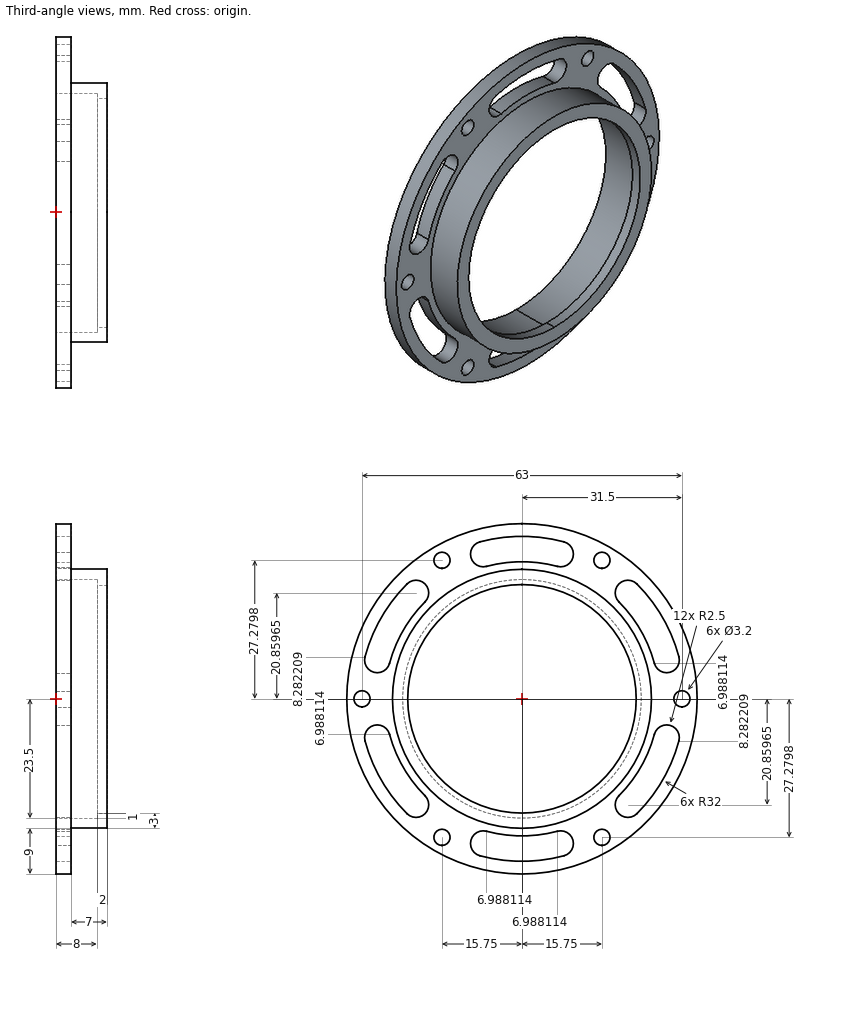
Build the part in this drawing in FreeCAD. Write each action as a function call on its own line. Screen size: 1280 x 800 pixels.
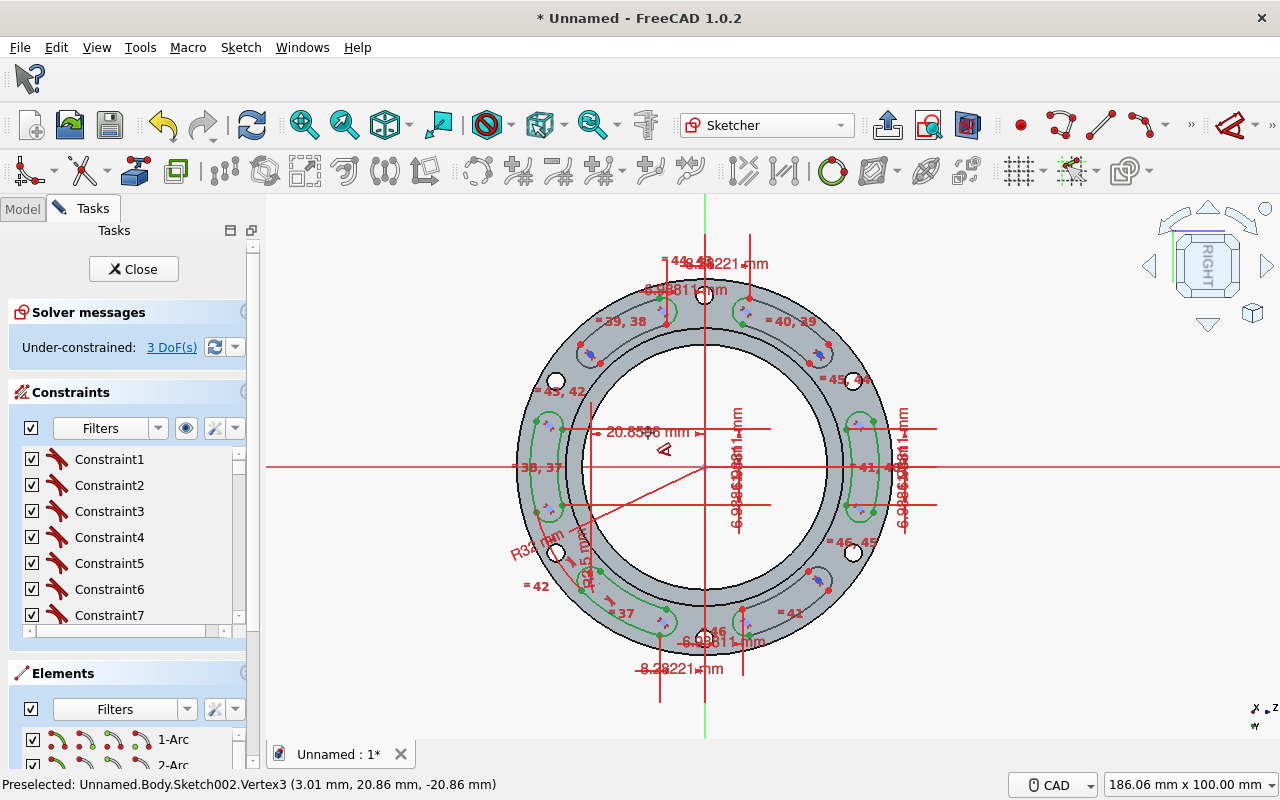
click(590, 354)
click(648, 501)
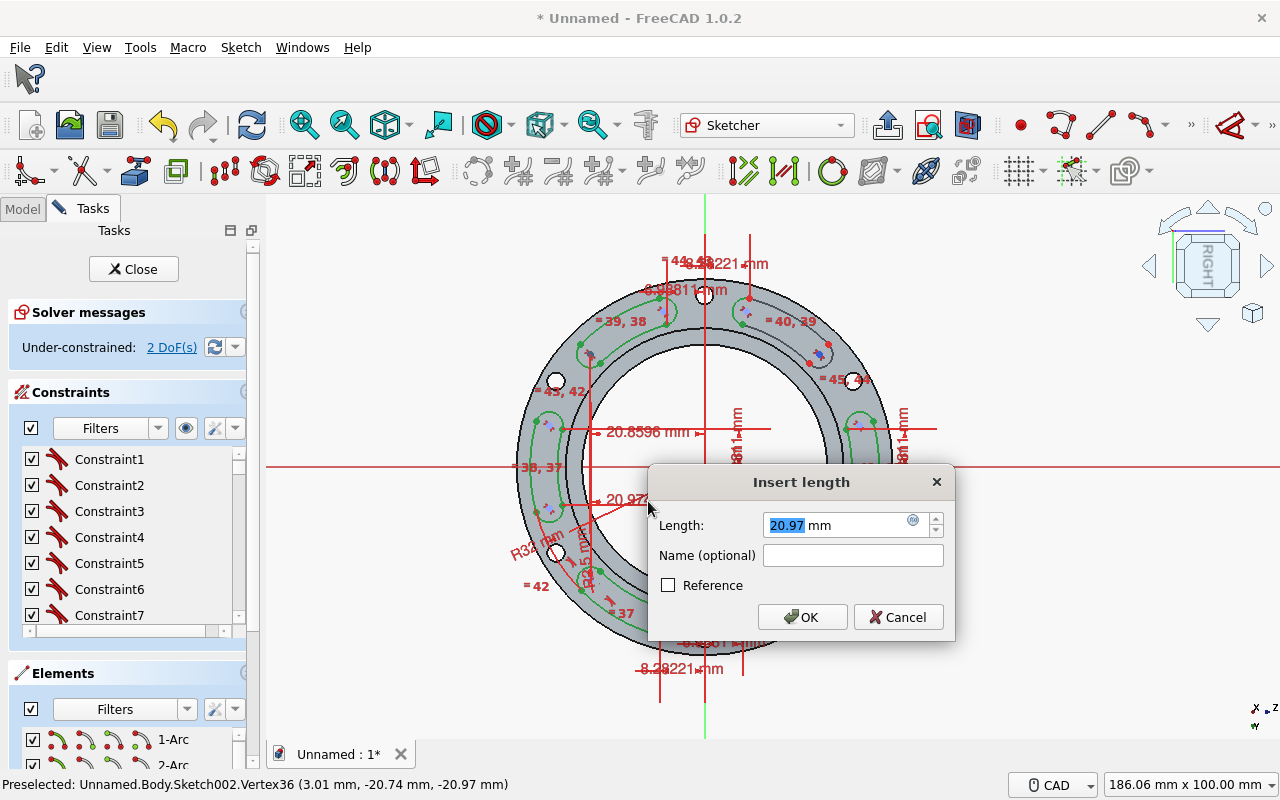
text(20.85965)
key(Return)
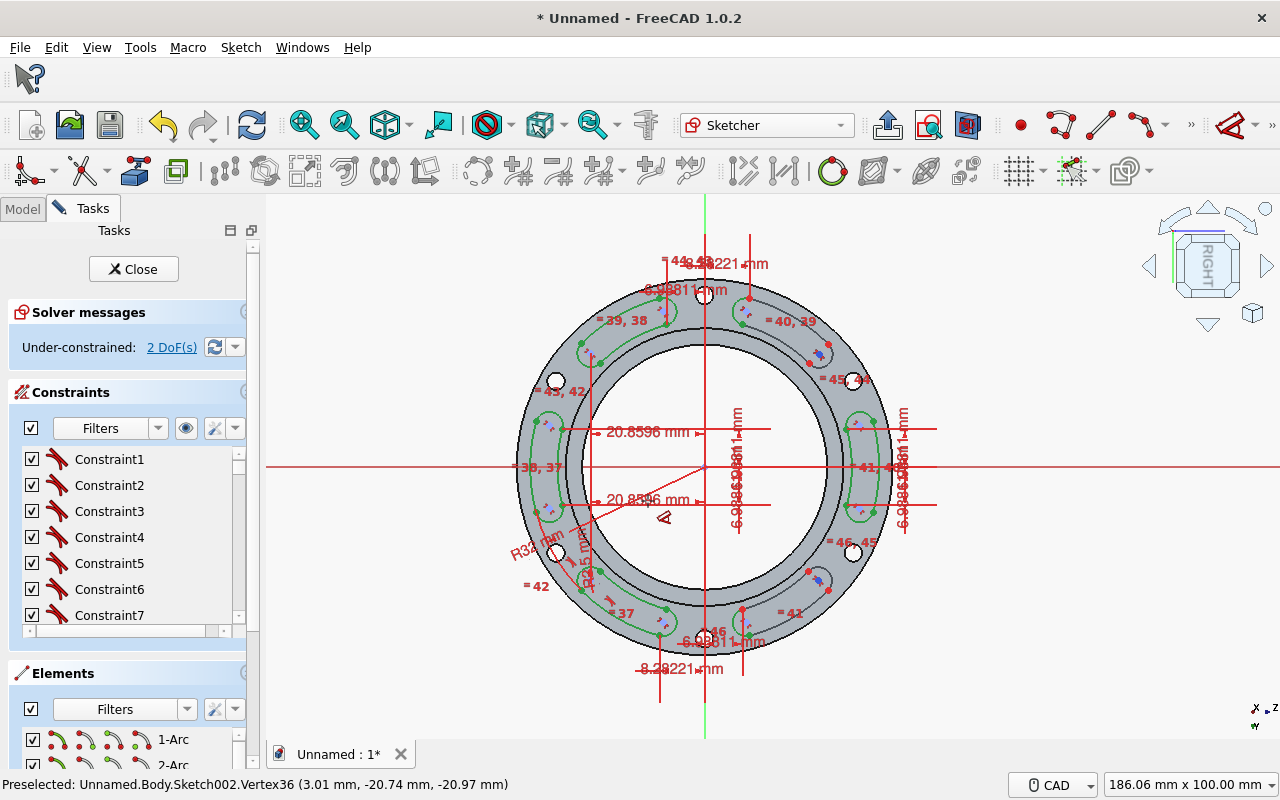
click(819, 354)
click(788, 296)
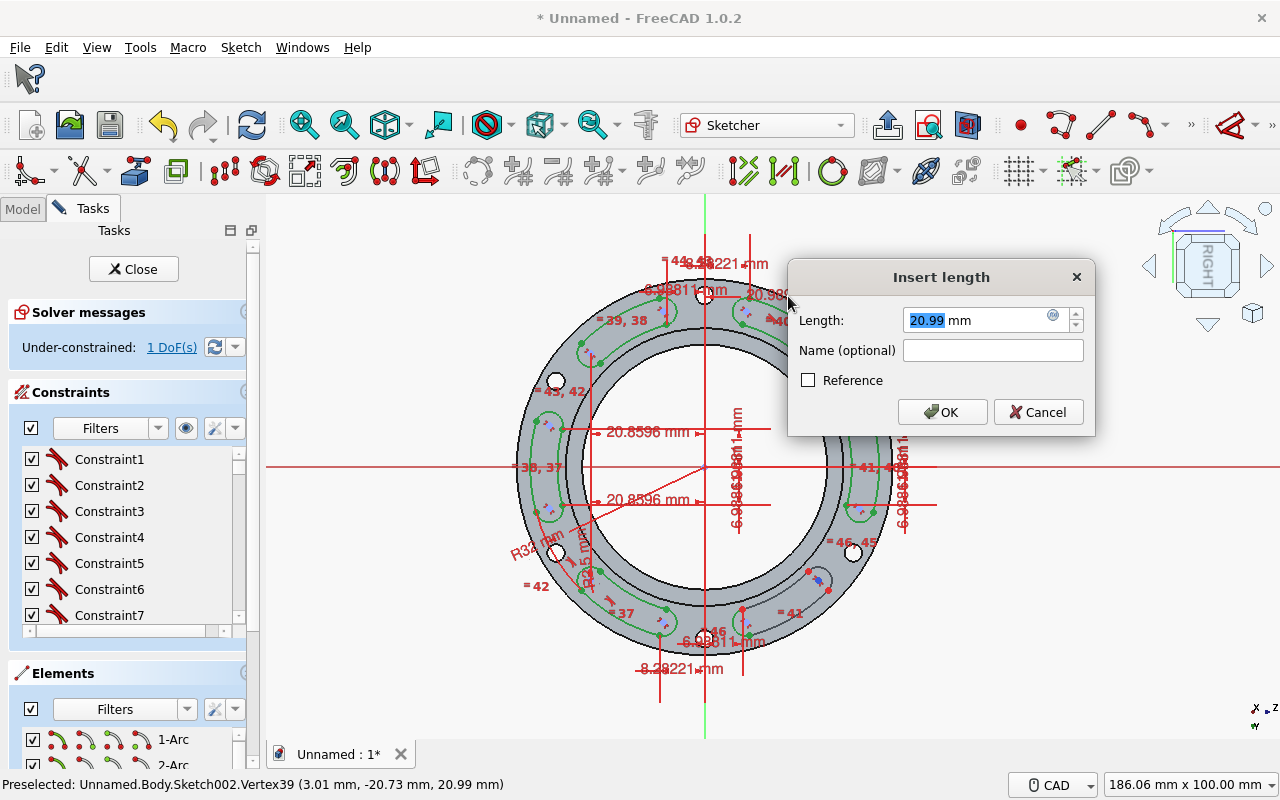
text(20.85965)
key(Return)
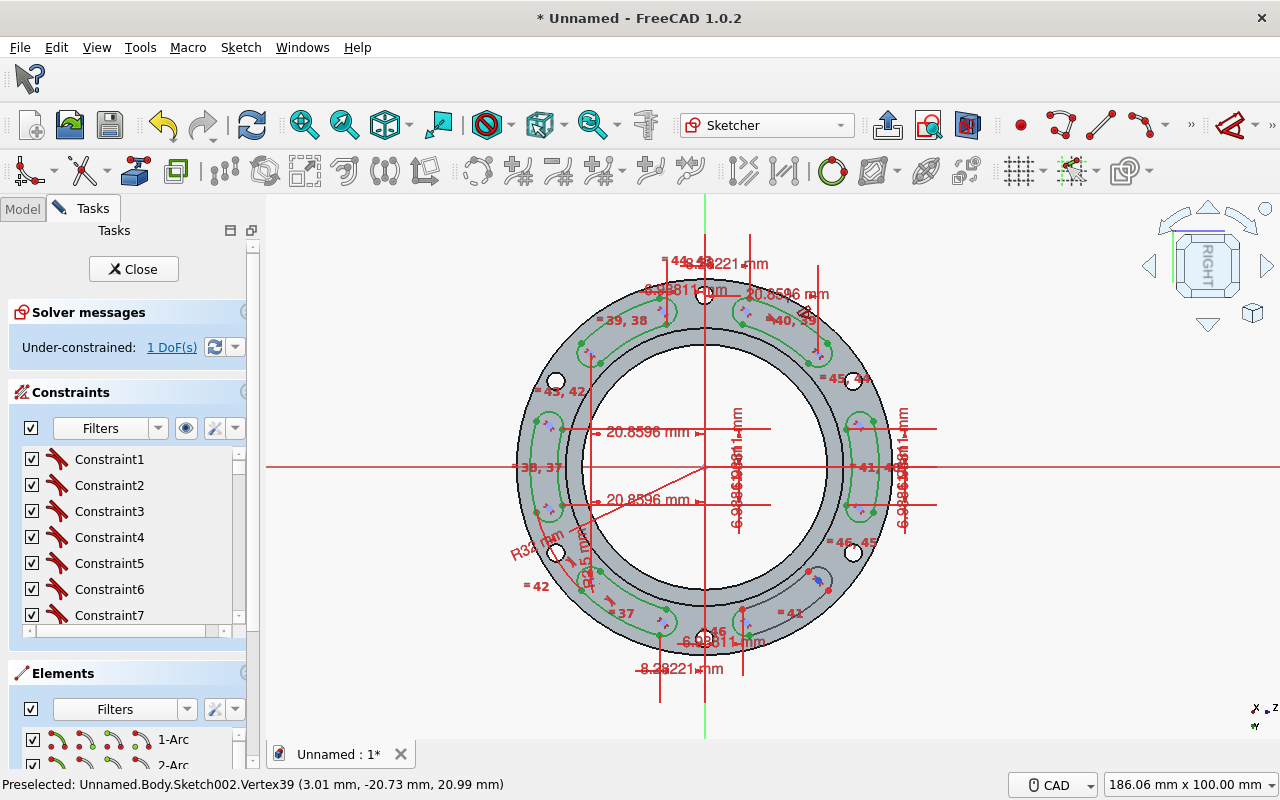
click(818, 581)
click(801, 639)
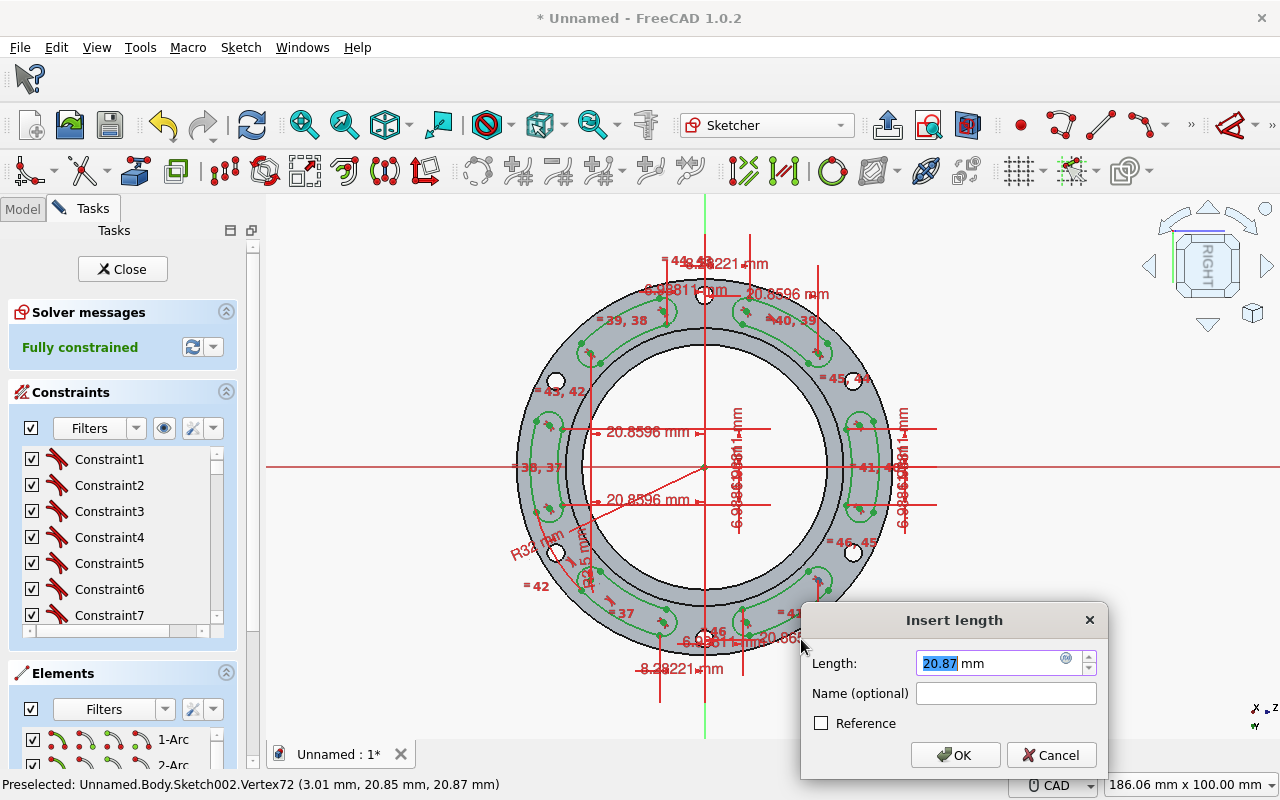
text(20.85965)
key(Return)
key(Escape)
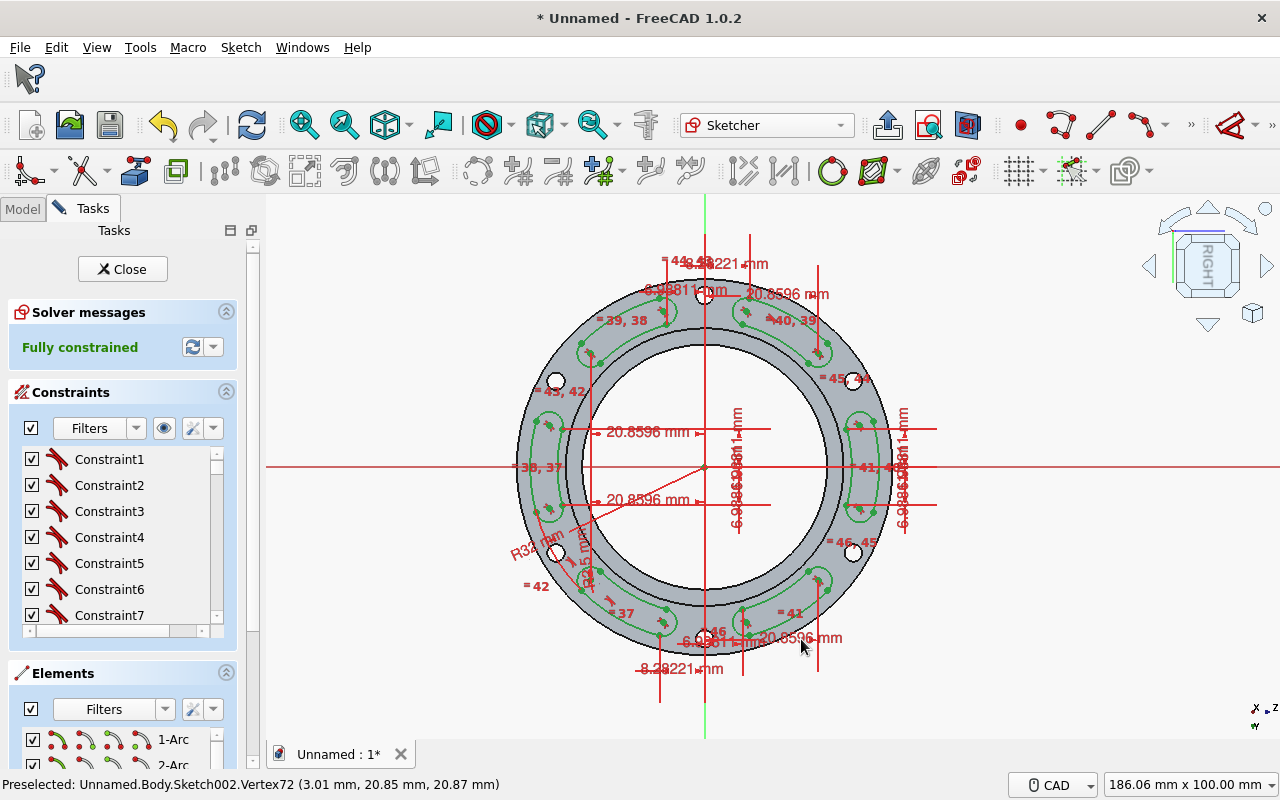
click(123, 269)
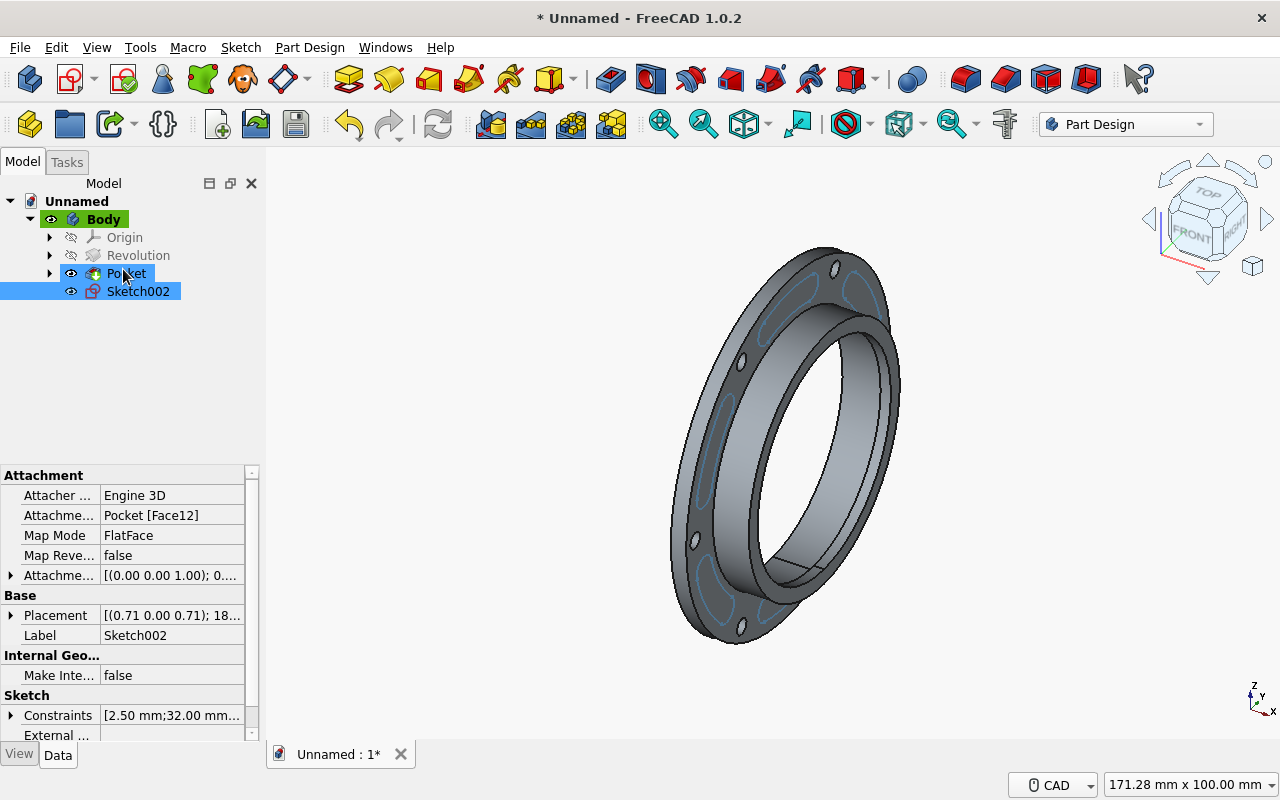
click(612, 80)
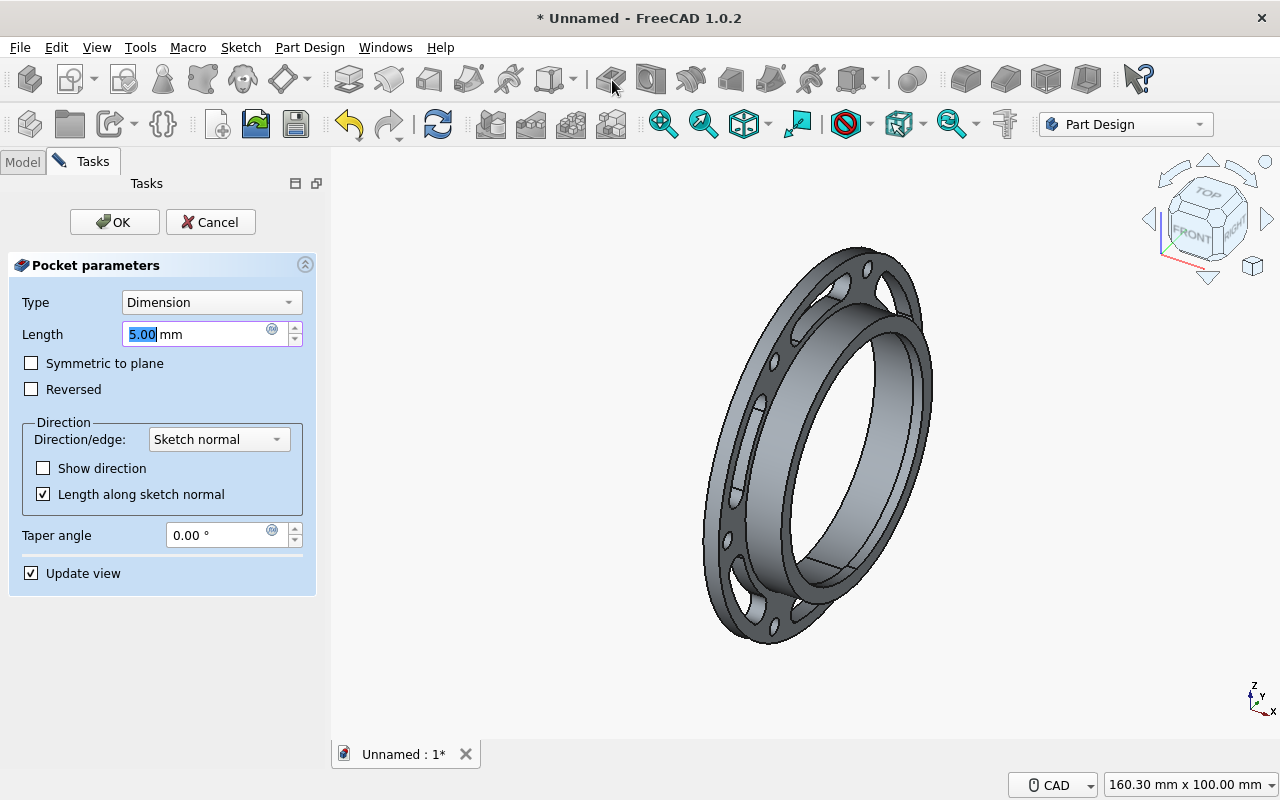
click(212, 302)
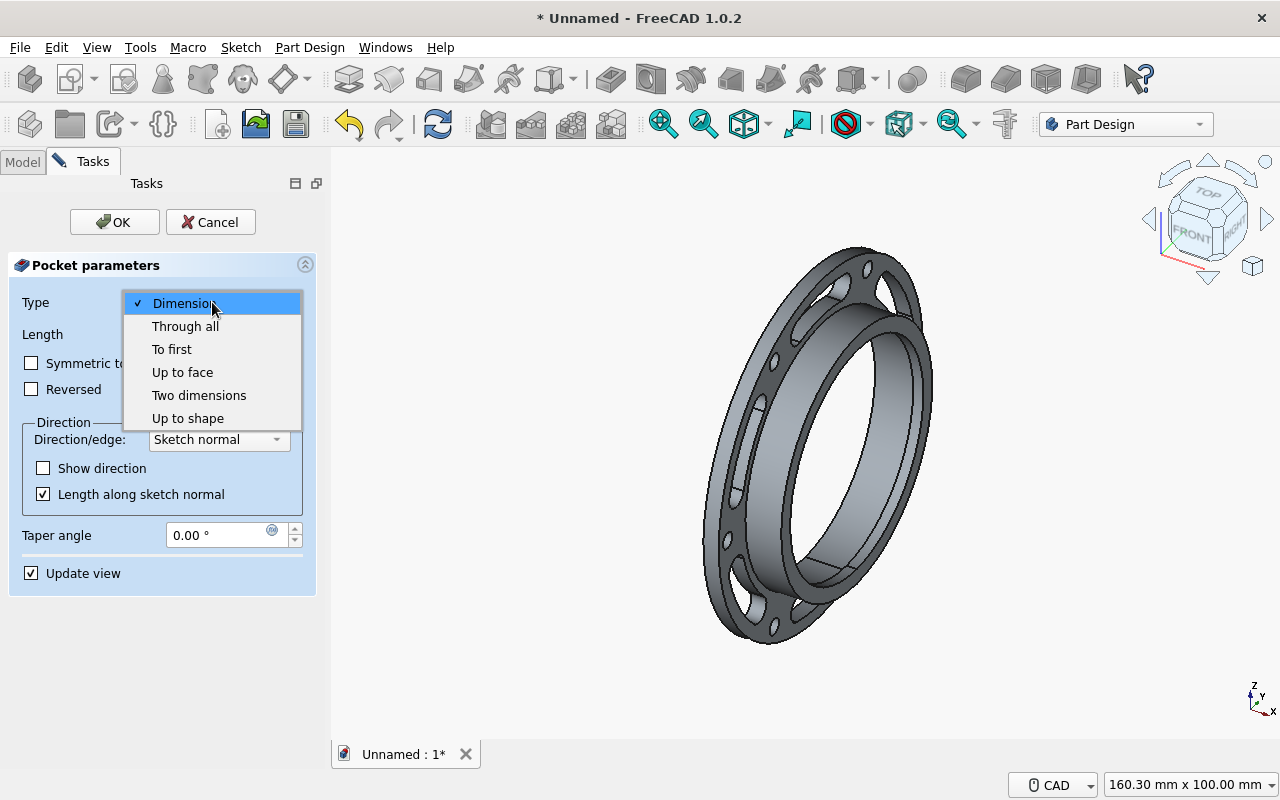
click(212, 326)